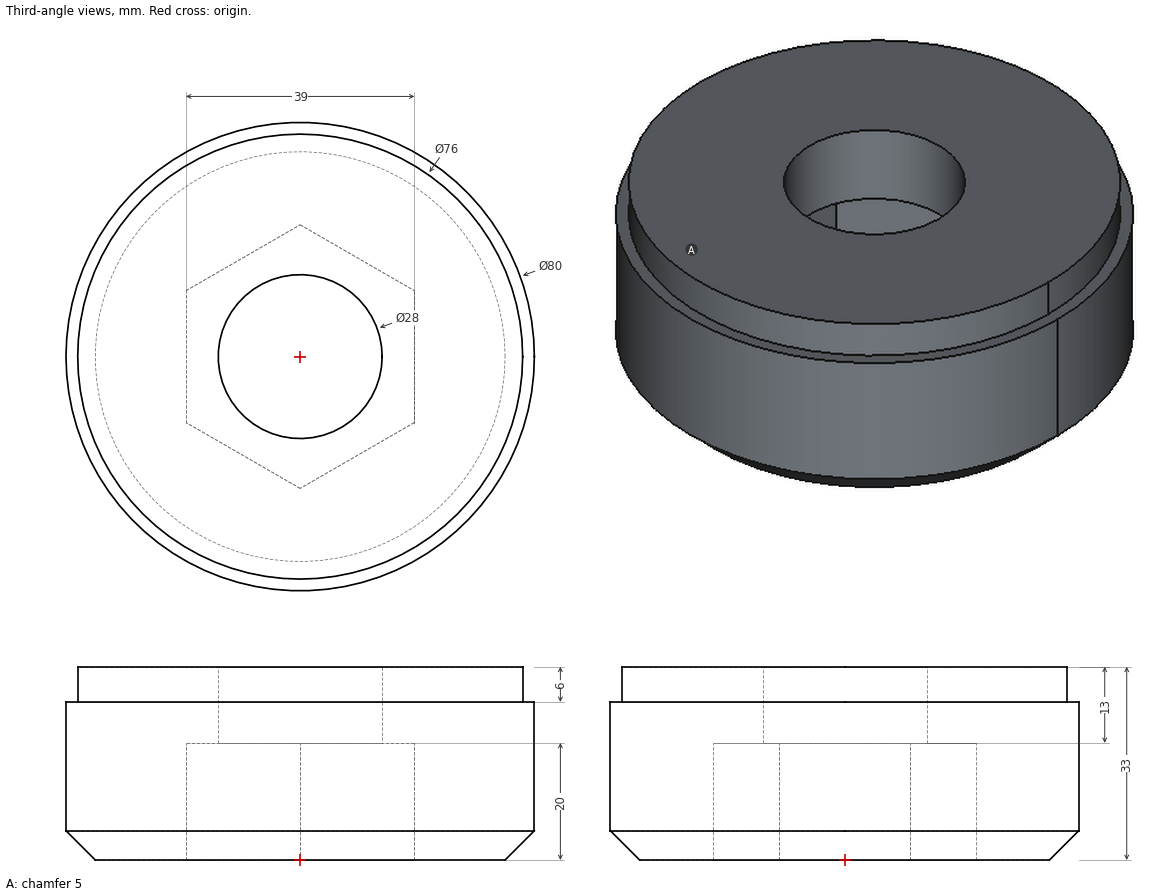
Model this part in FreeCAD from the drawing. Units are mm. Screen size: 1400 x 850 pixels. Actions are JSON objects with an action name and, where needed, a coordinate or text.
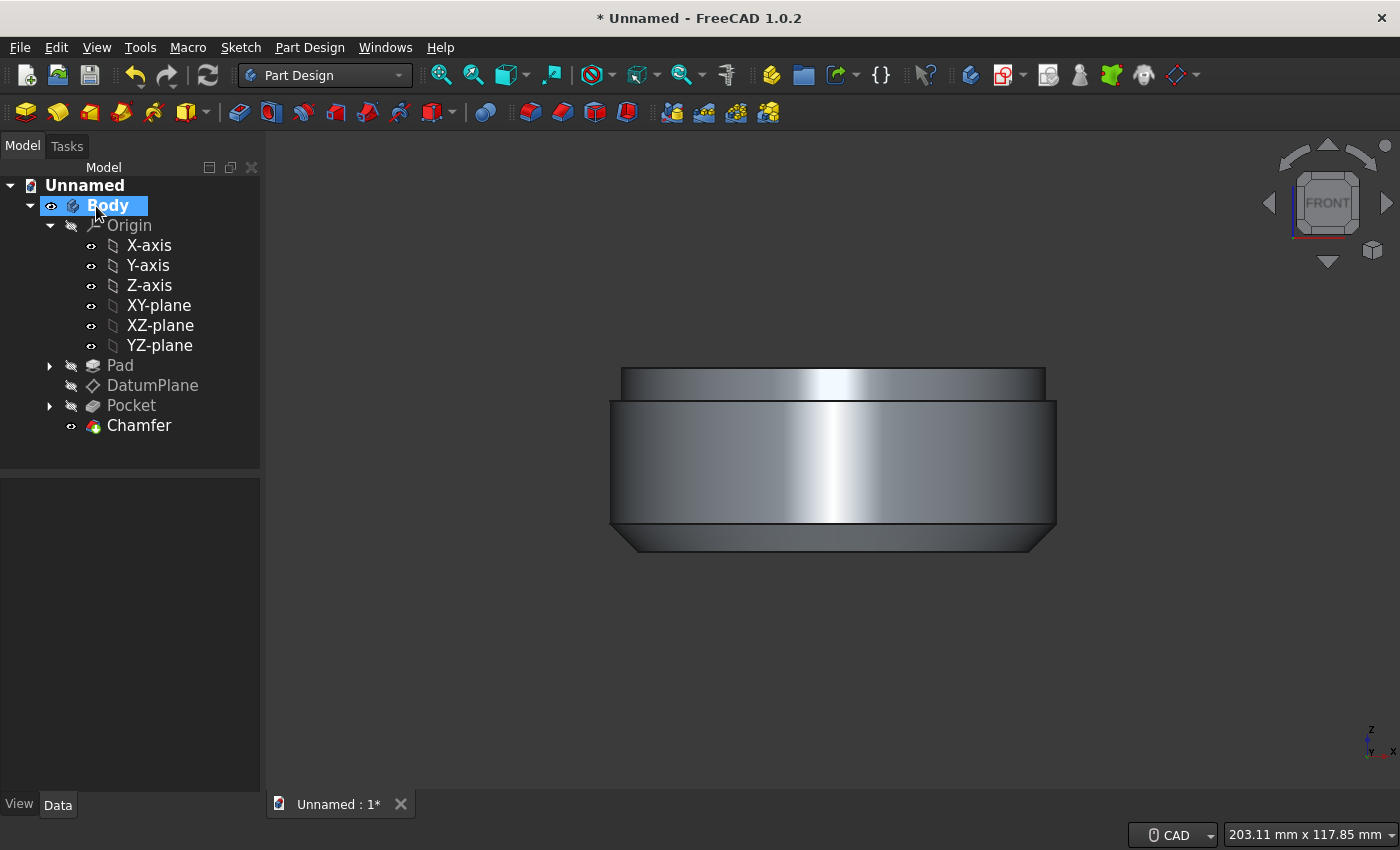
{"action": "left_click", "coordinate": [442, 76]}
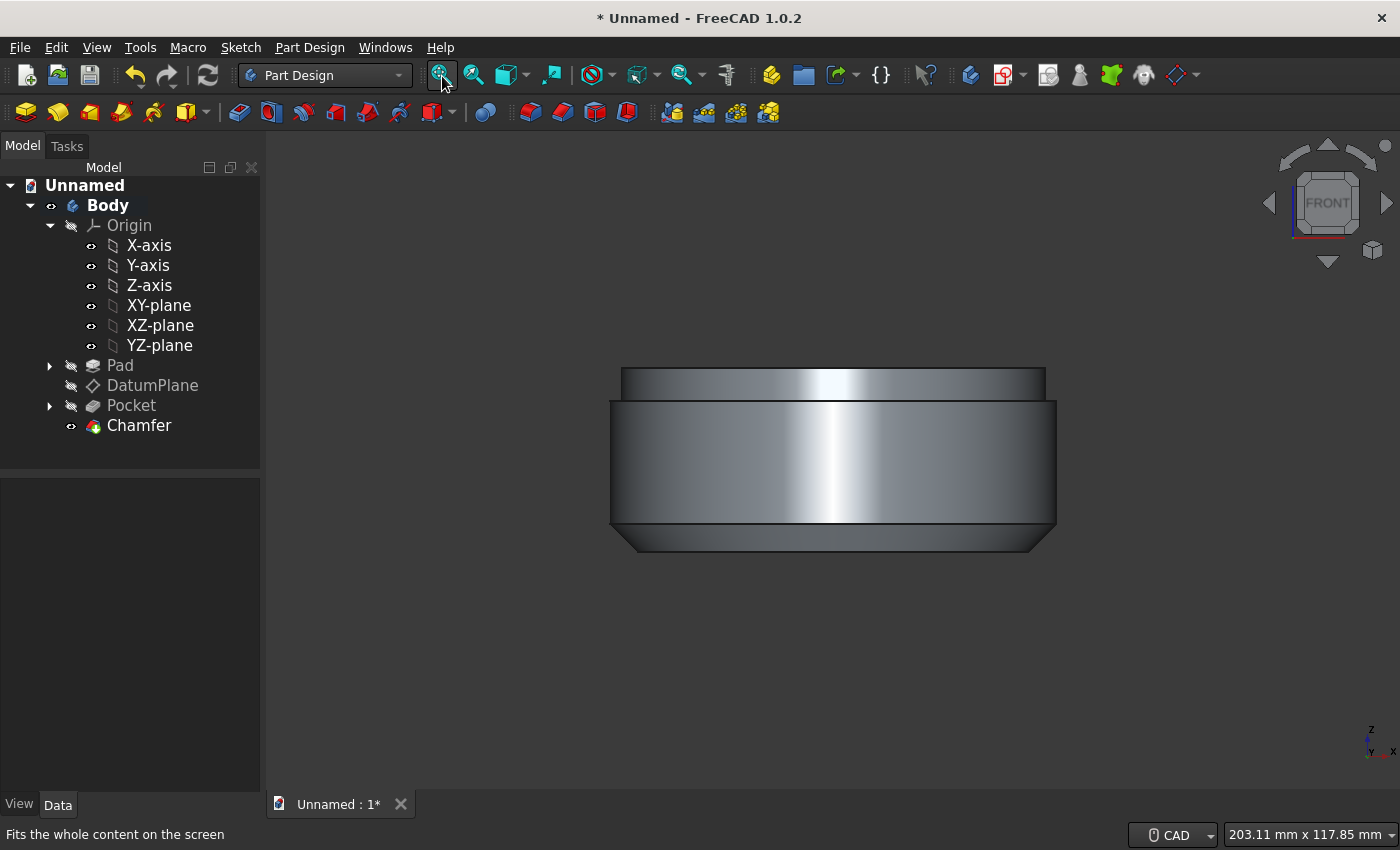
{"action": "key", "text": "0"}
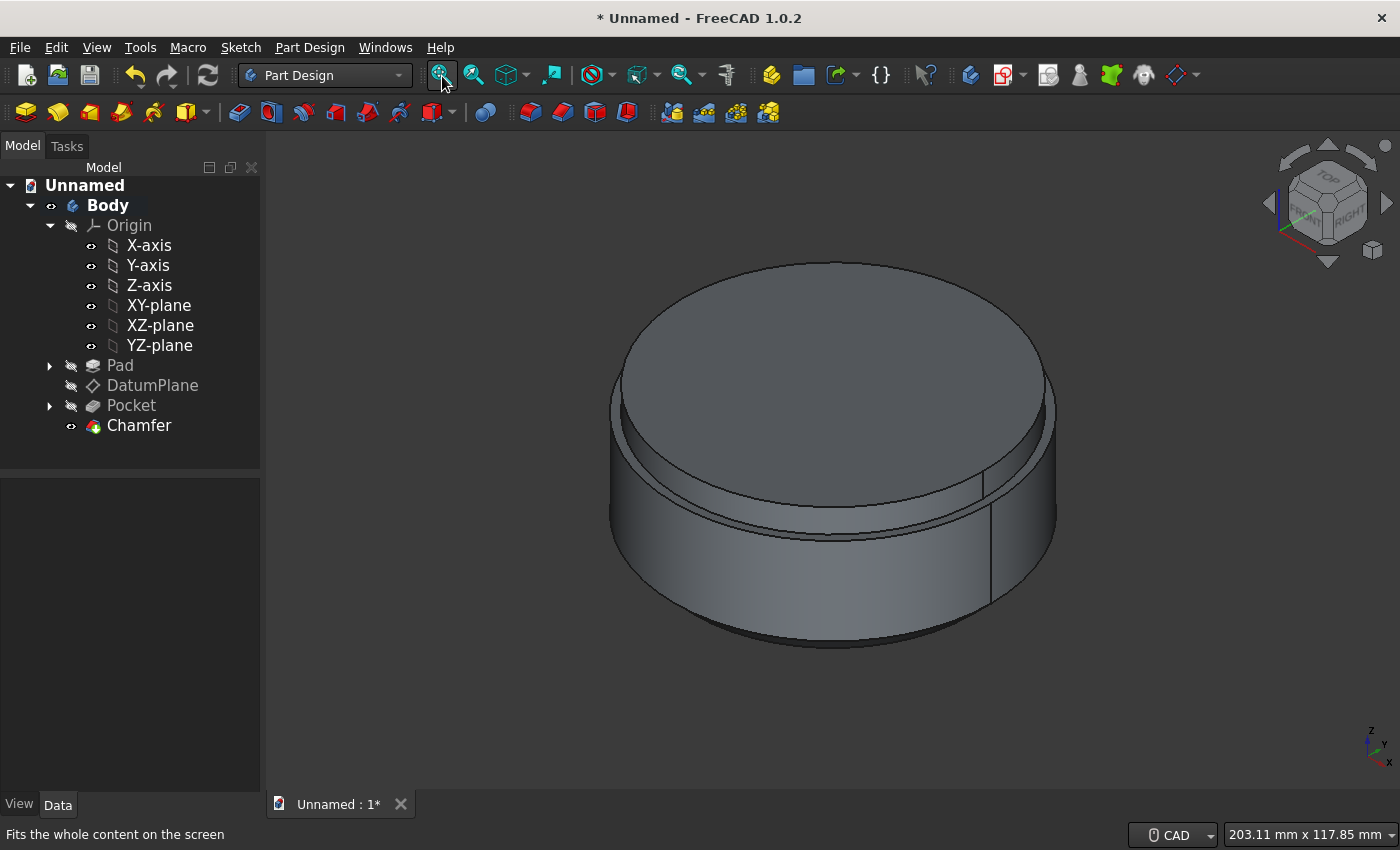
{"action": "left_click", "coordinate": [833, 384]}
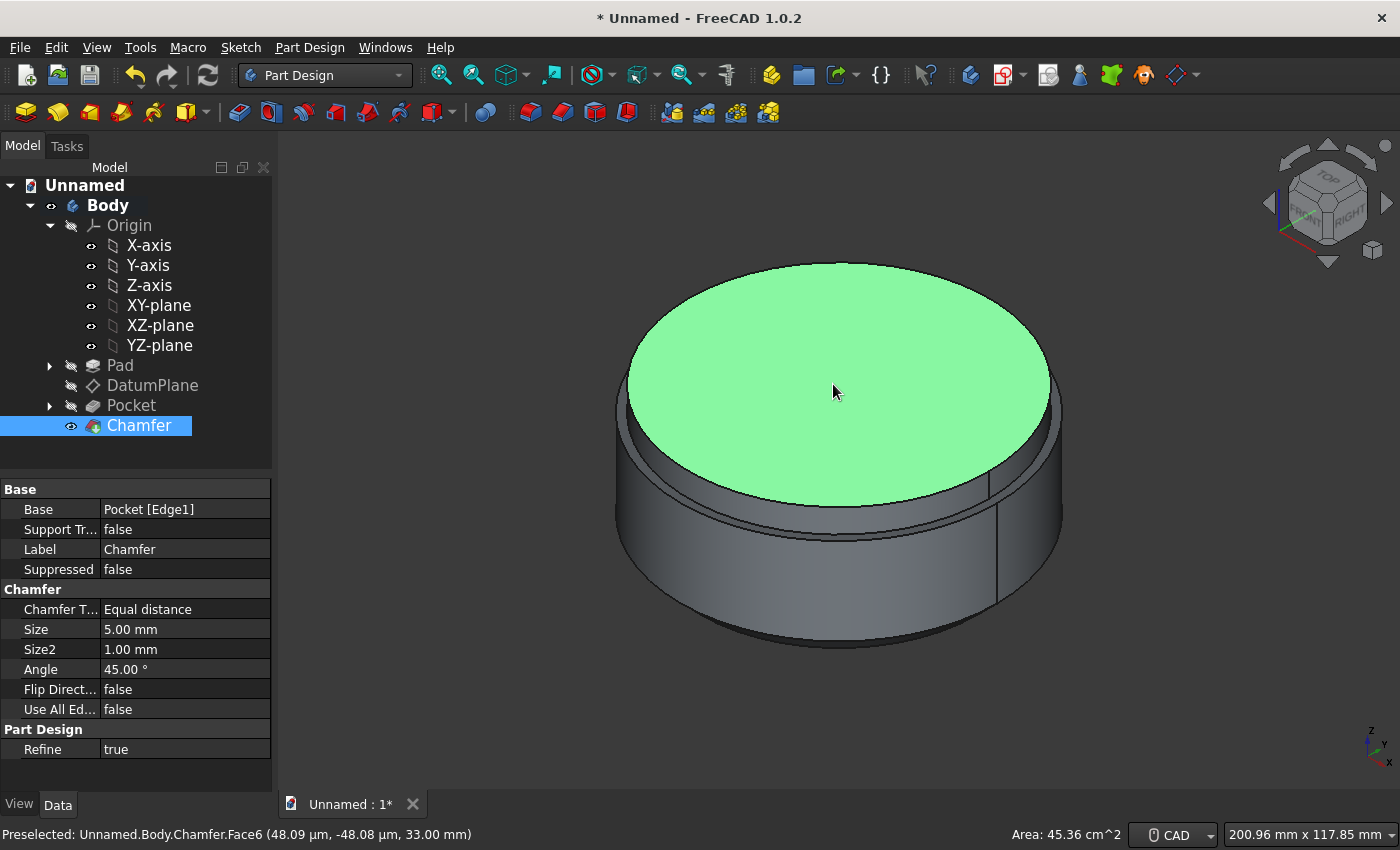
{"action": "left_click", "coordinate": [1004, 76]}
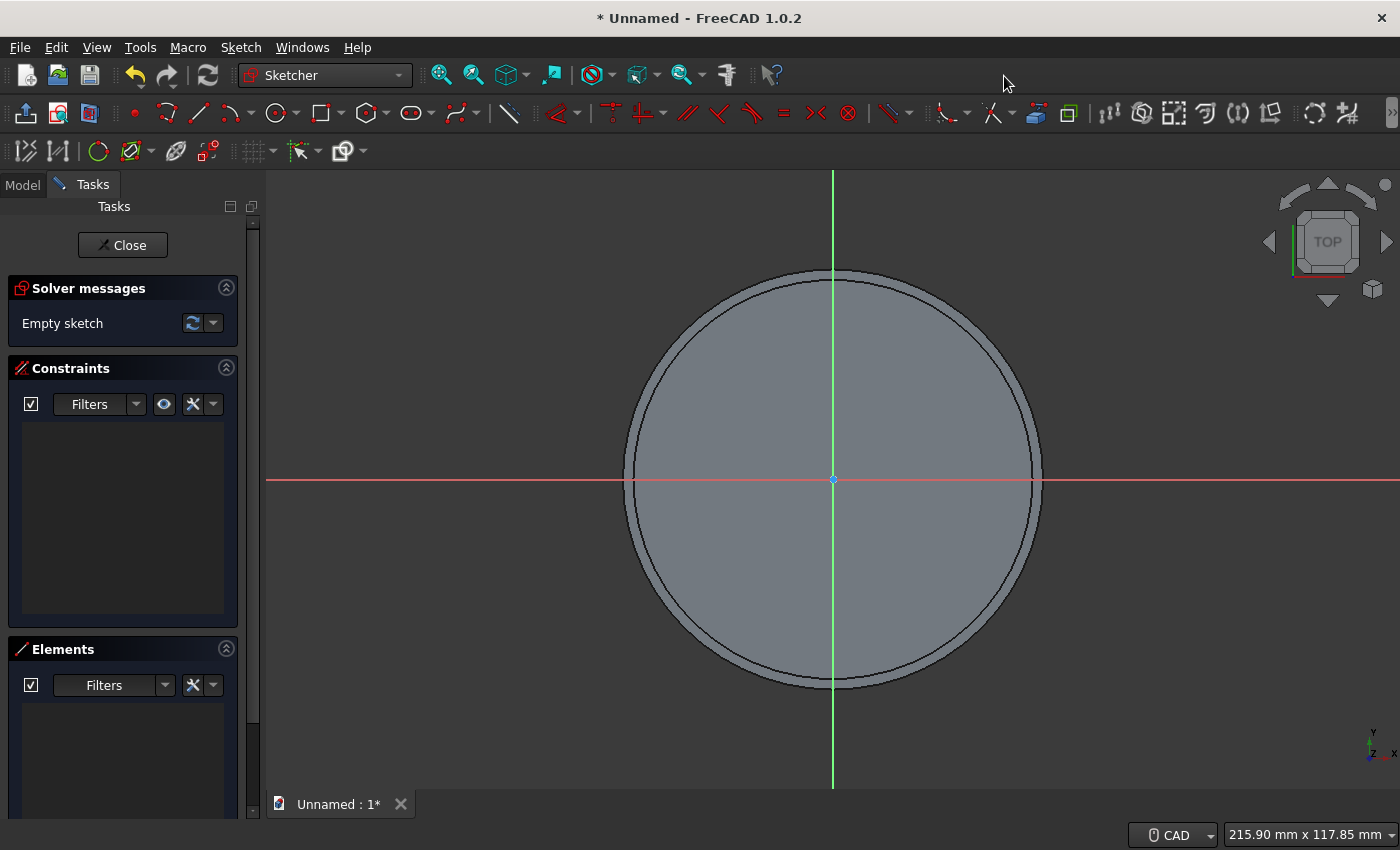
{"action": "scroll", "coordinate": [873, 480], "scroll_direction": "up", "scroll_amount": 5}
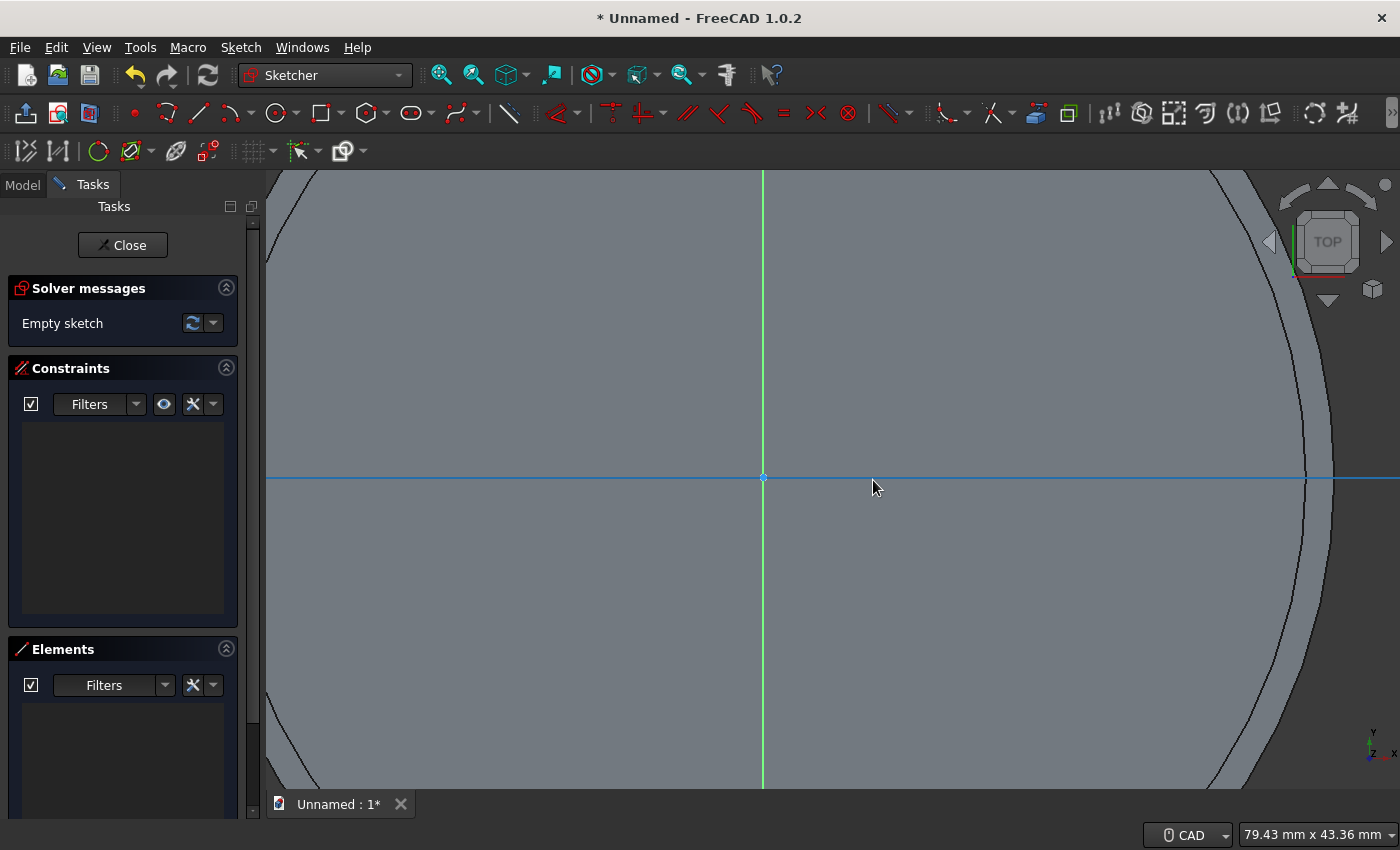
{"action": "left_click", "coordinate": [276, 114]}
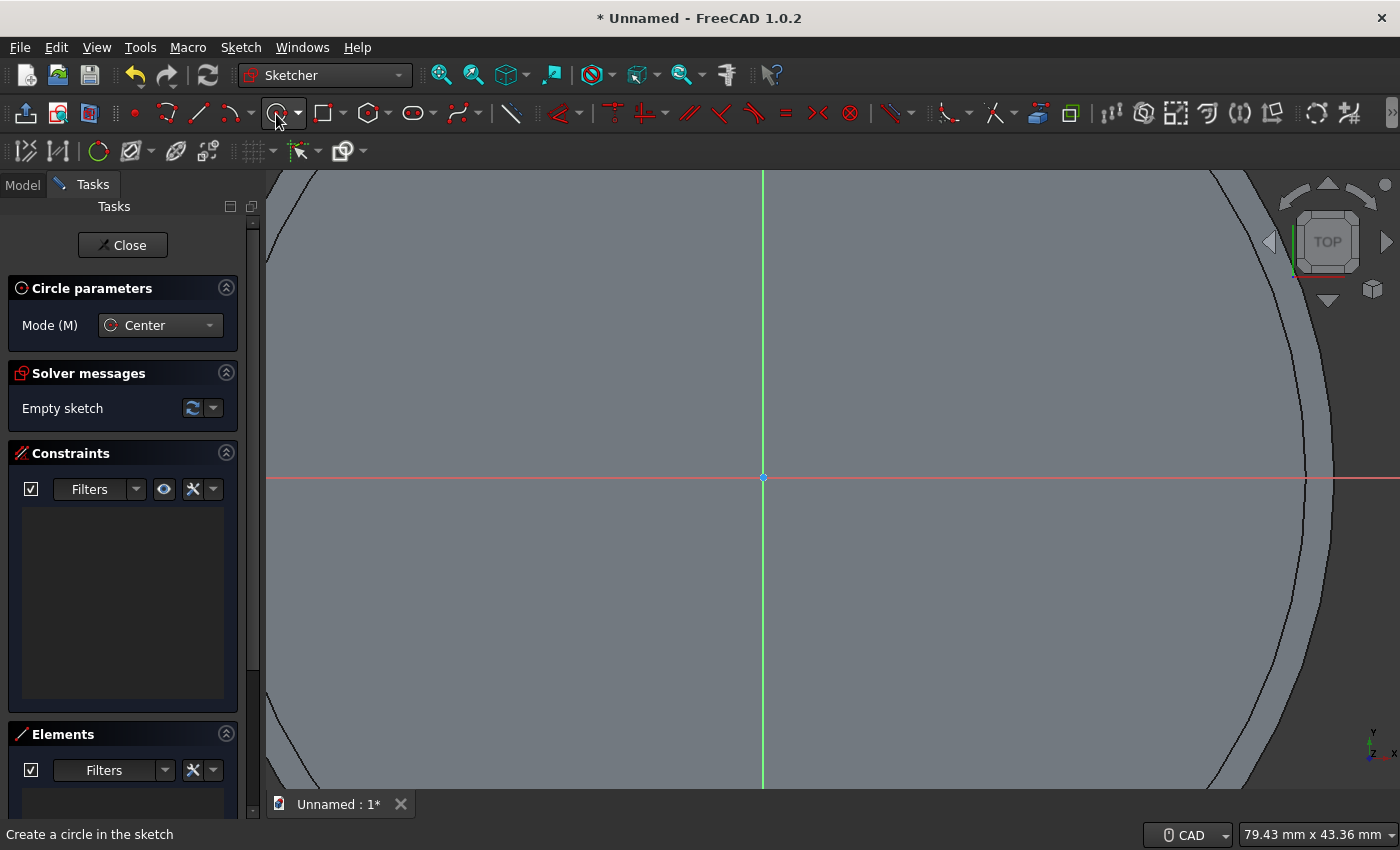
{"action": "left_click", "coordinate": [763, 478]}
{"action": "left_click", "coordinate": [905, 336]}
{"action": "key", "text": "Escape"}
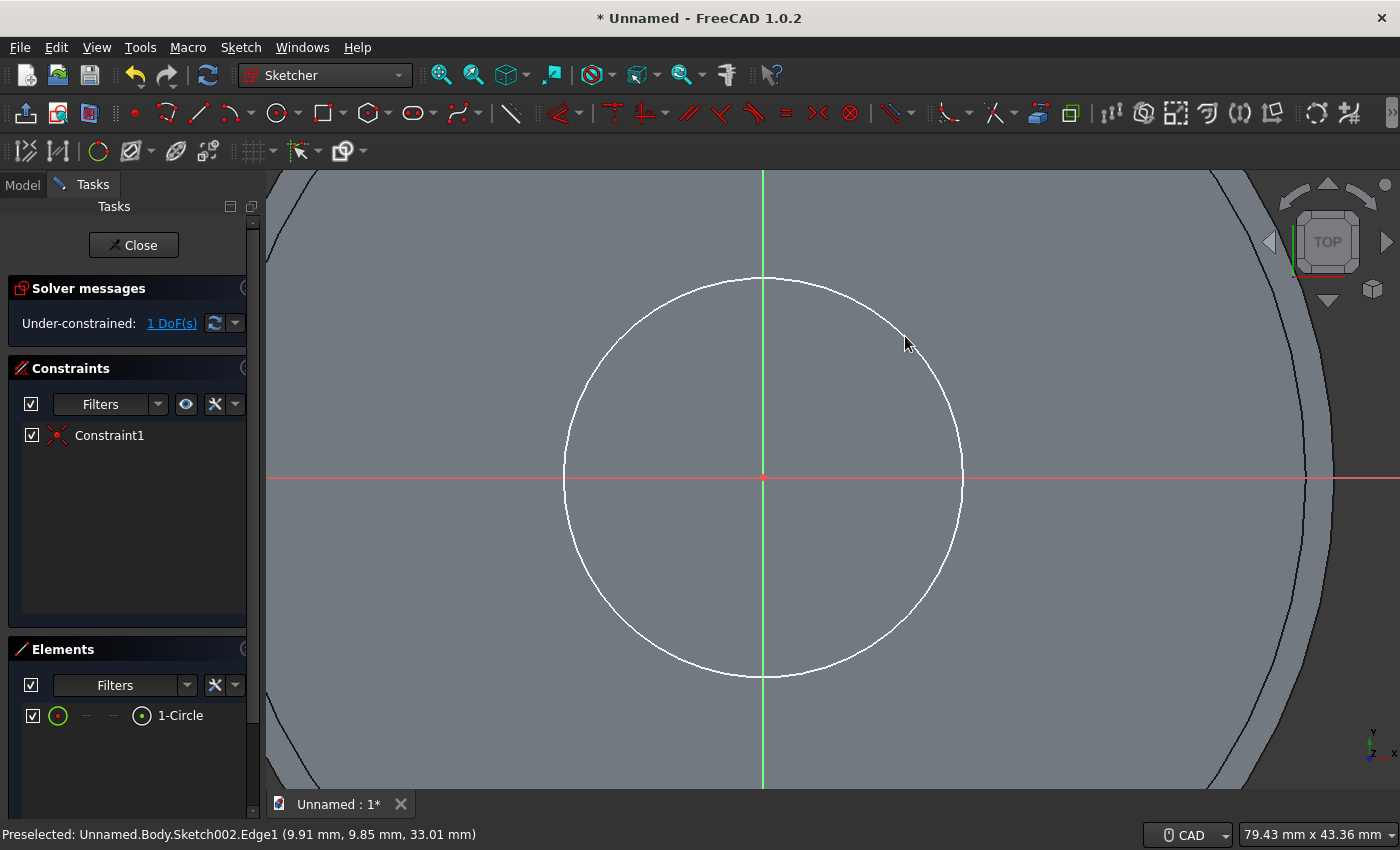
{"action": "left_click", "coordinate": [558, 114]}